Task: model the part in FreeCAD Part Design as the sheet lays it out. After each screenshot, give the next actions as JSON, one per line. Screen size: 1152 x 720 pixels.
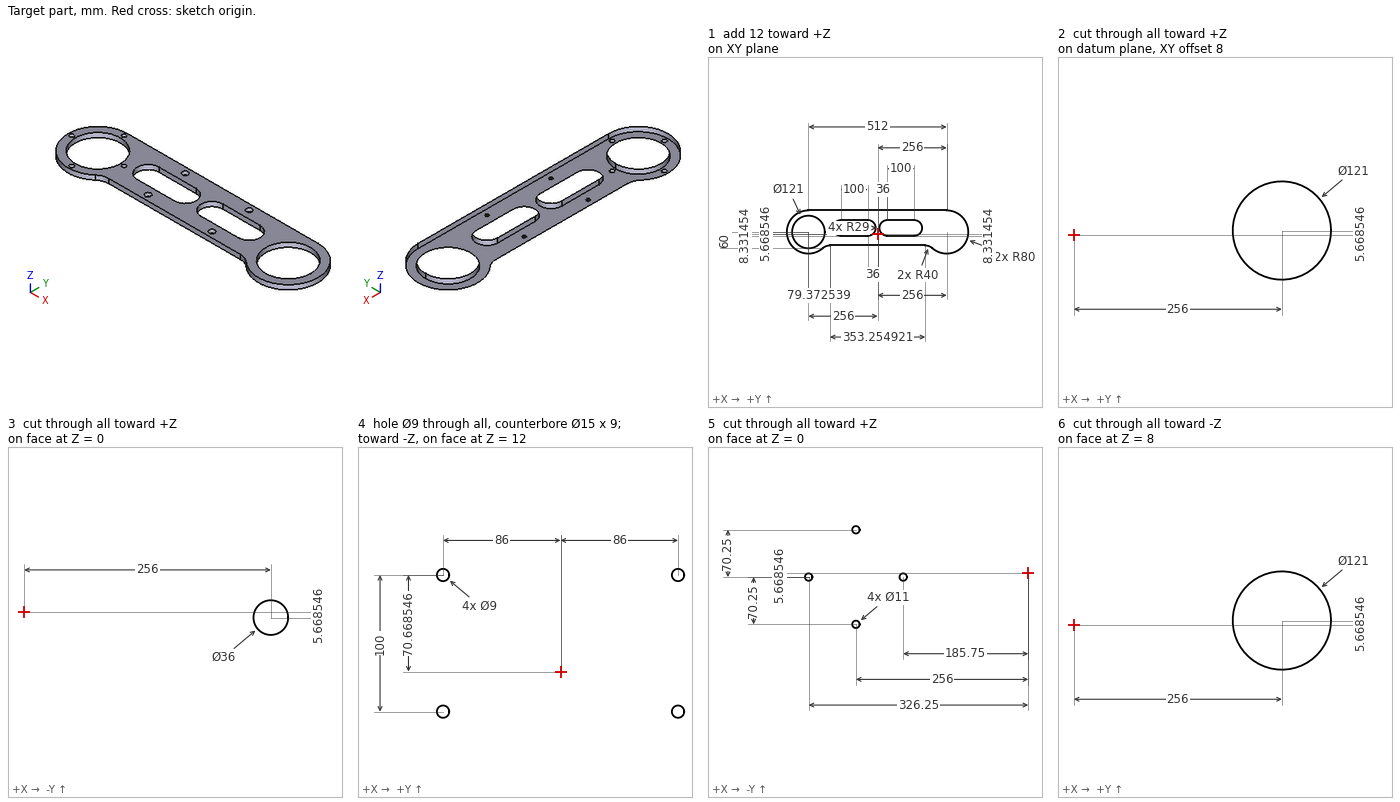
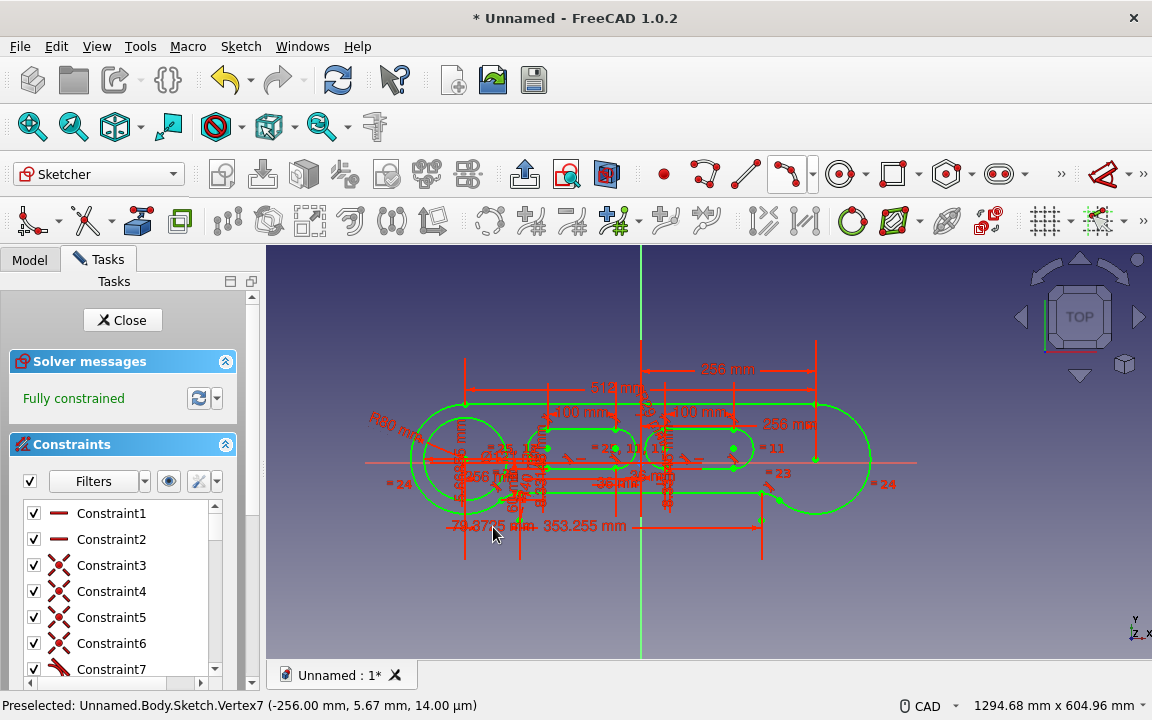
{"action": "left_click", "coordinate": [123, 320]}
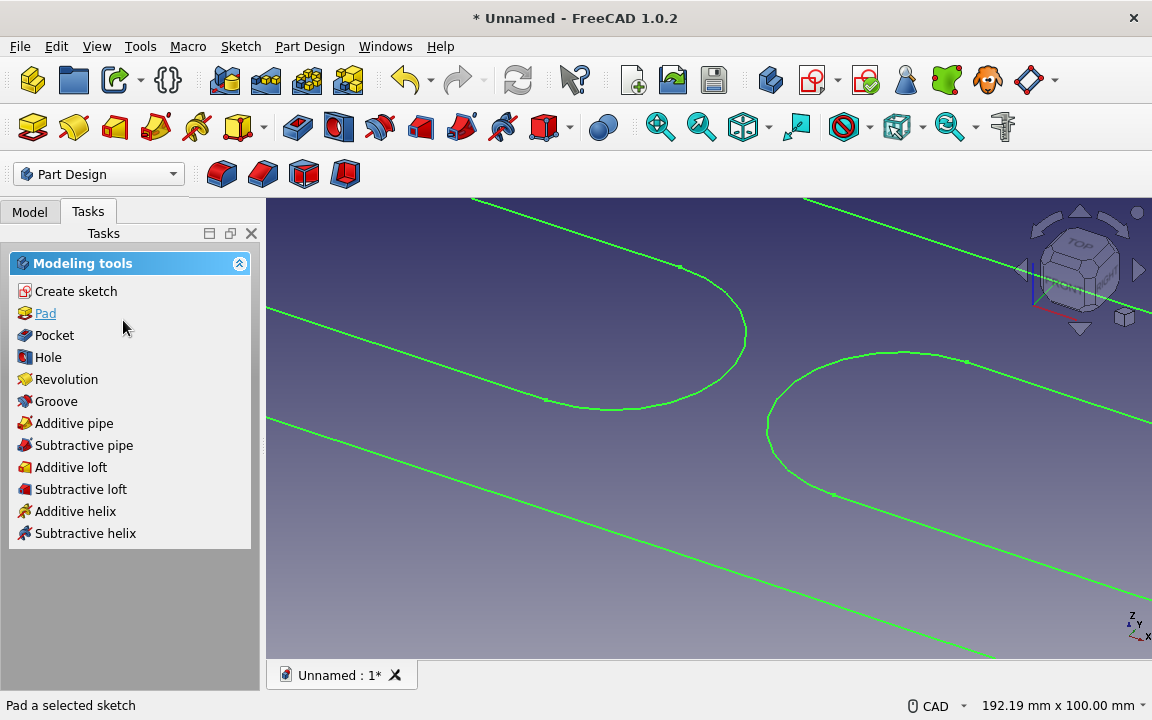
{"action": "left_click", "coordinate": [33, 128]}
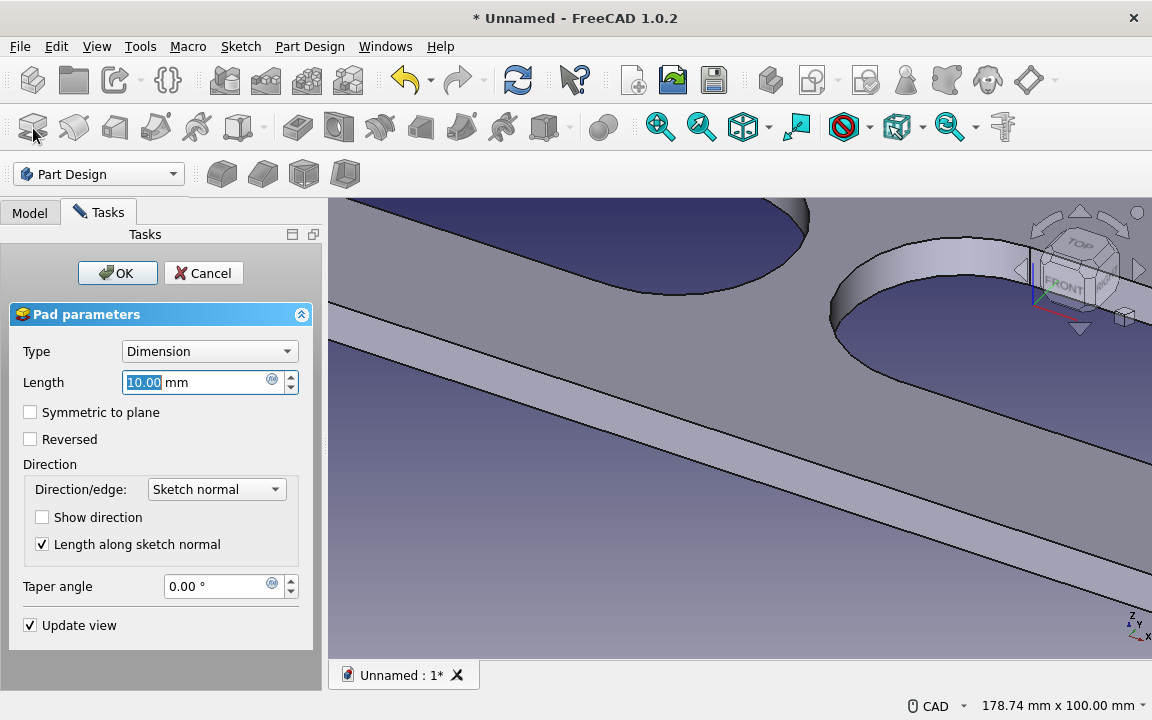
{"action": "type", "text": "12"}
{"action": "key", "text": "Tab"}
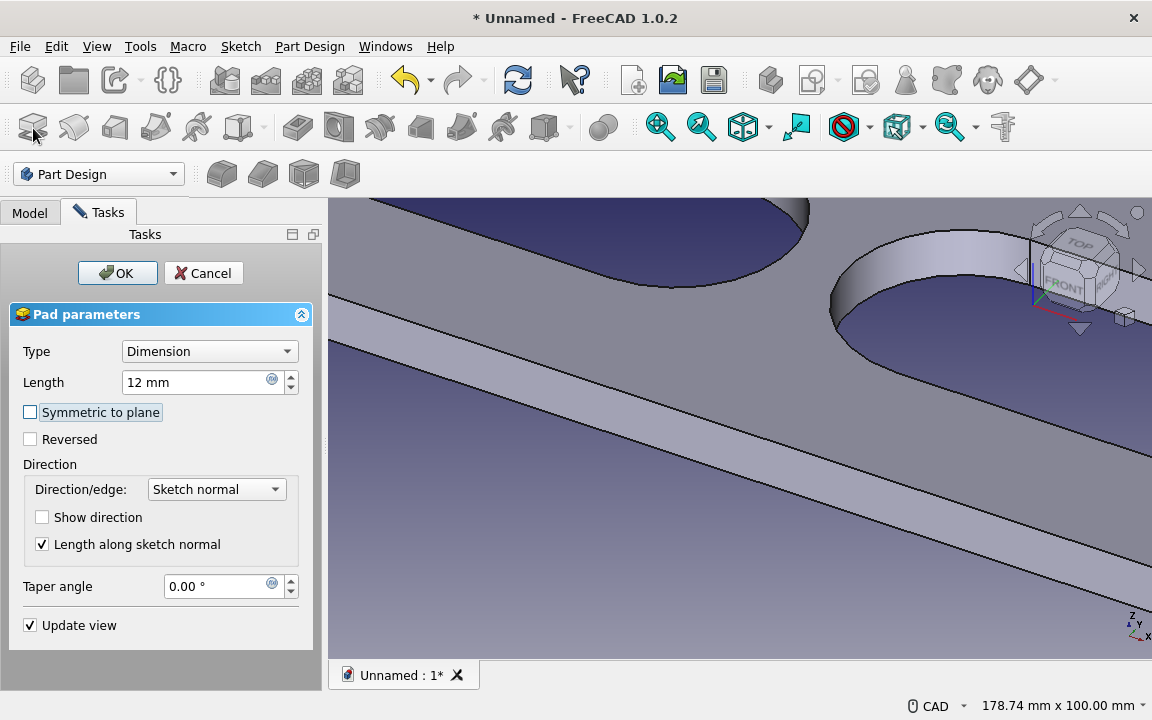
{"action": "left_click", "coordinate": [118, 273]}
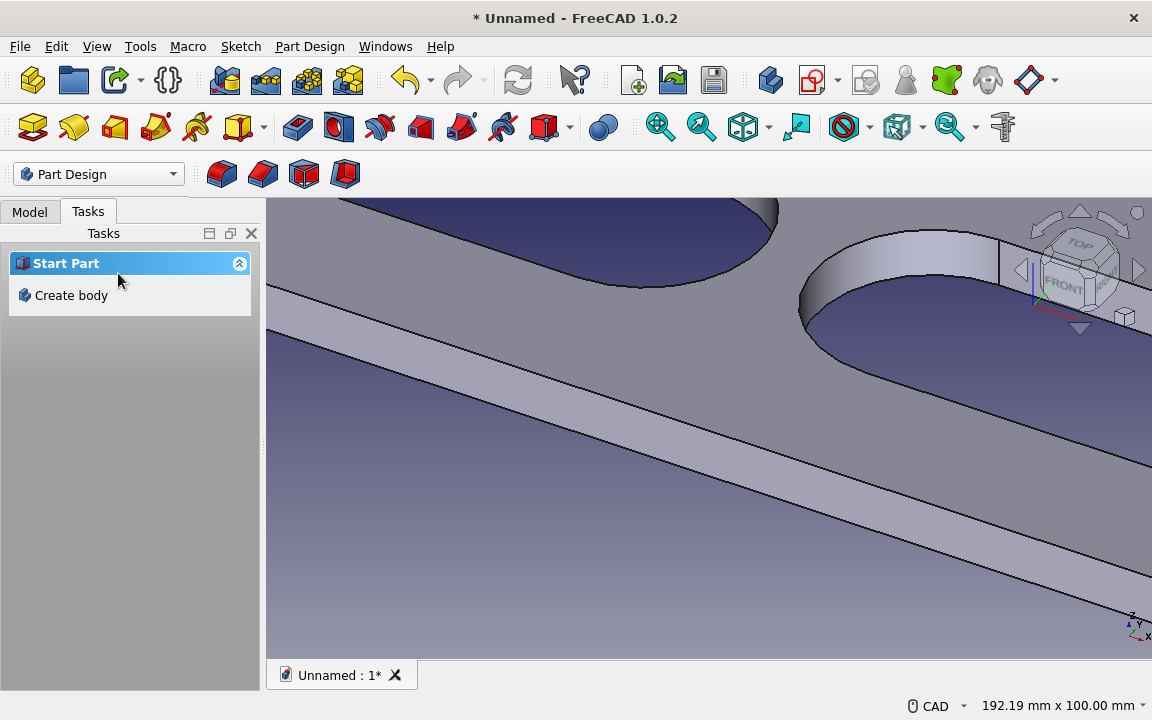
{"action": "left_click", "coordinate": [661, 128]}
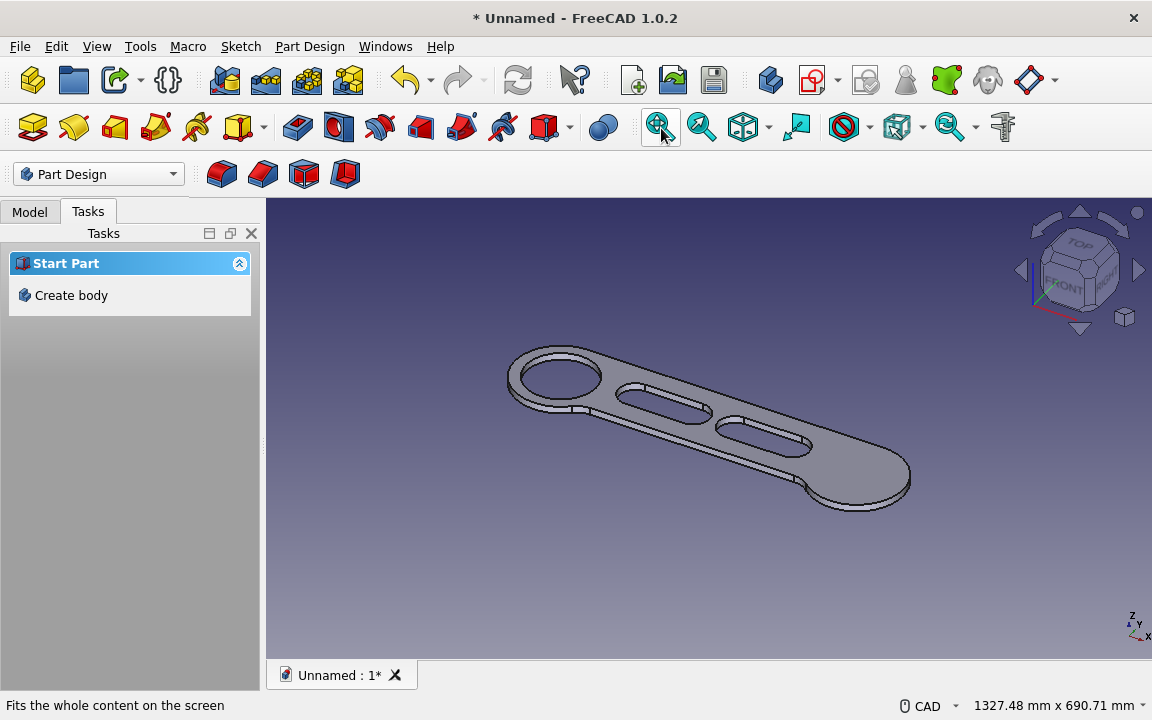
{"action": "left_click", "coordinate": [30, 212]}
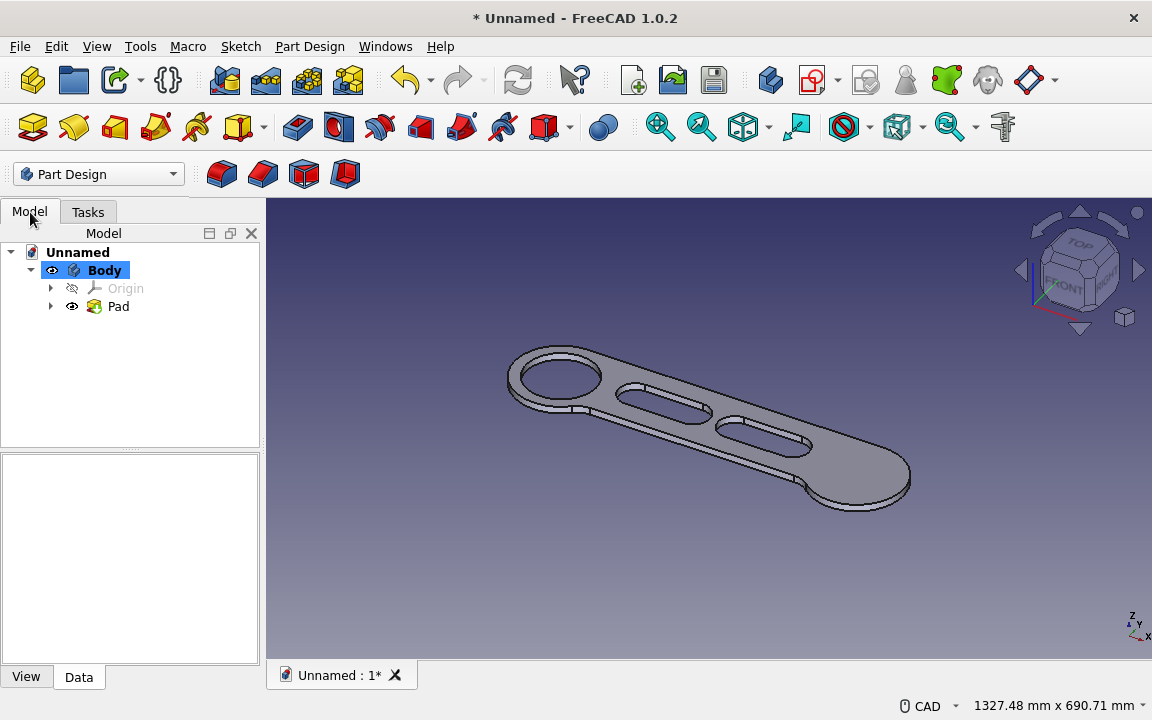
{"action": "left_click", "coordinate": [51, 288]}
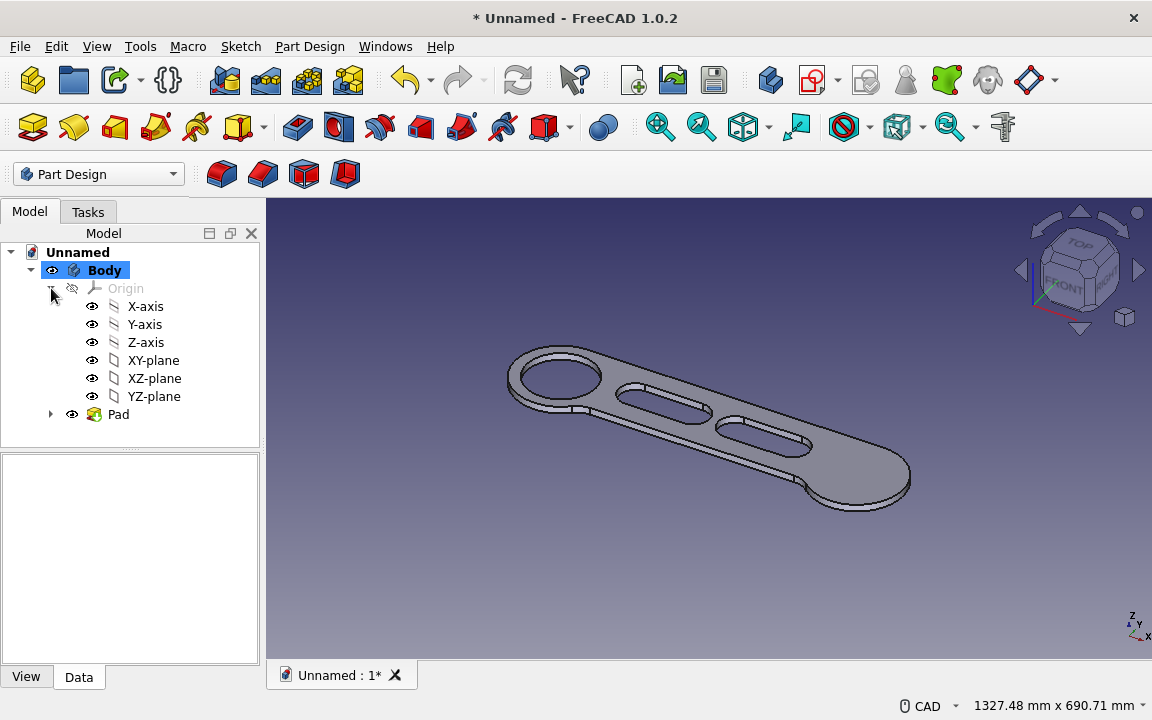
{"action": "left_click", "coordinate": [137, 360]}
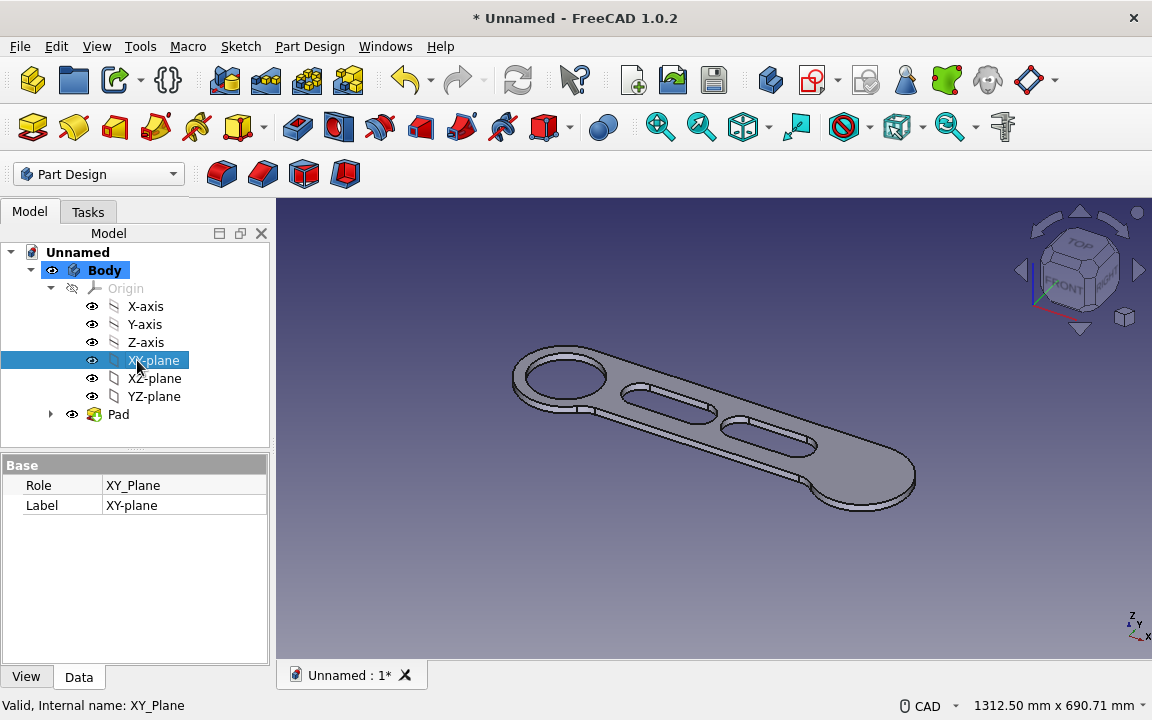
{"action": "left_click", "coordinate": [1028, 80]}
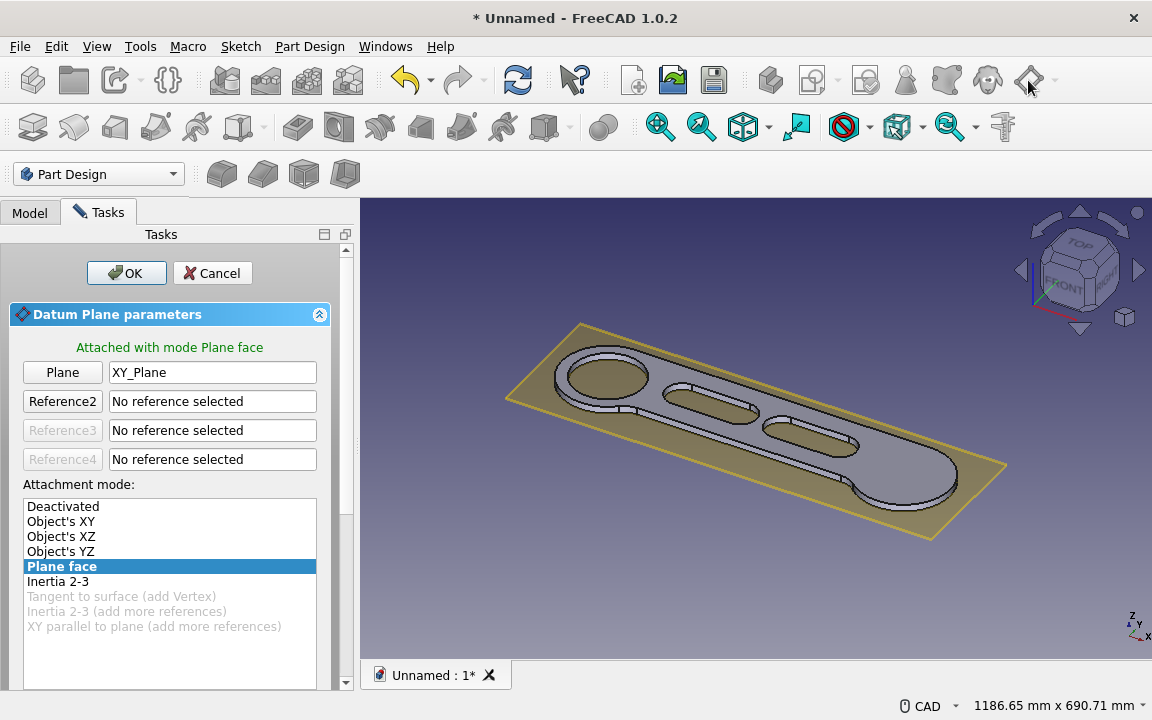
{"action": "scroll", "coordinate": [346, 467], "scroll_direction": "down", "scroll_amount": 4}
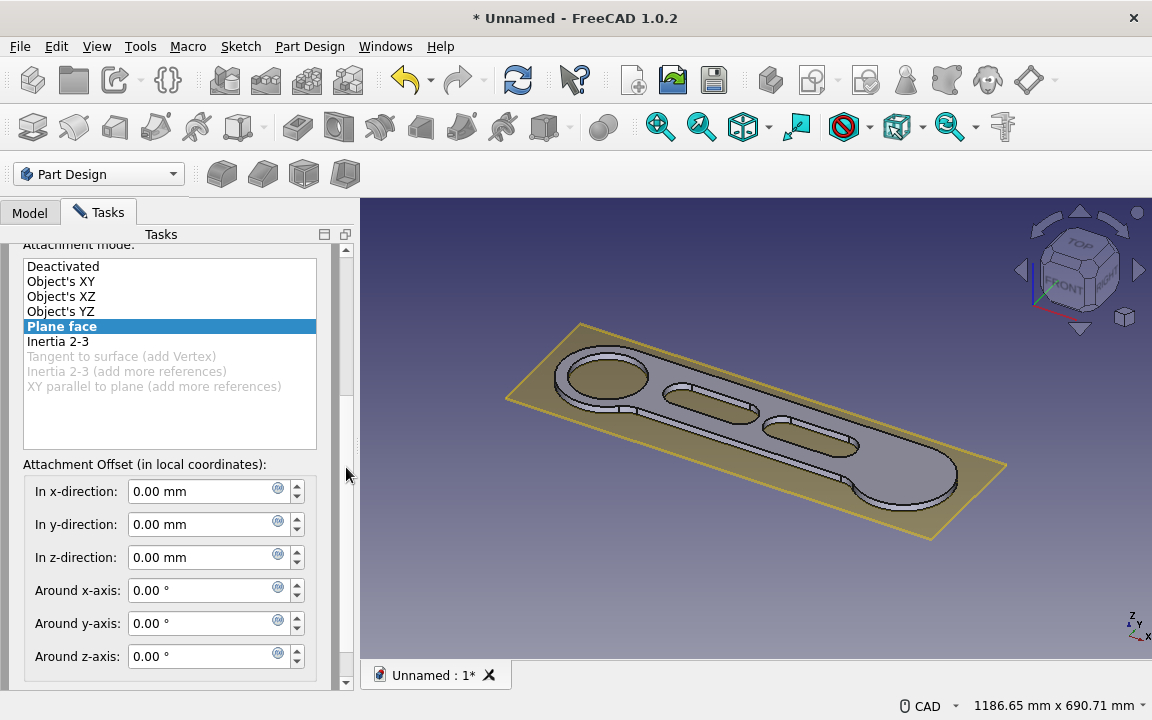
{"action": "triple_click", "coordinate": [210, 558]}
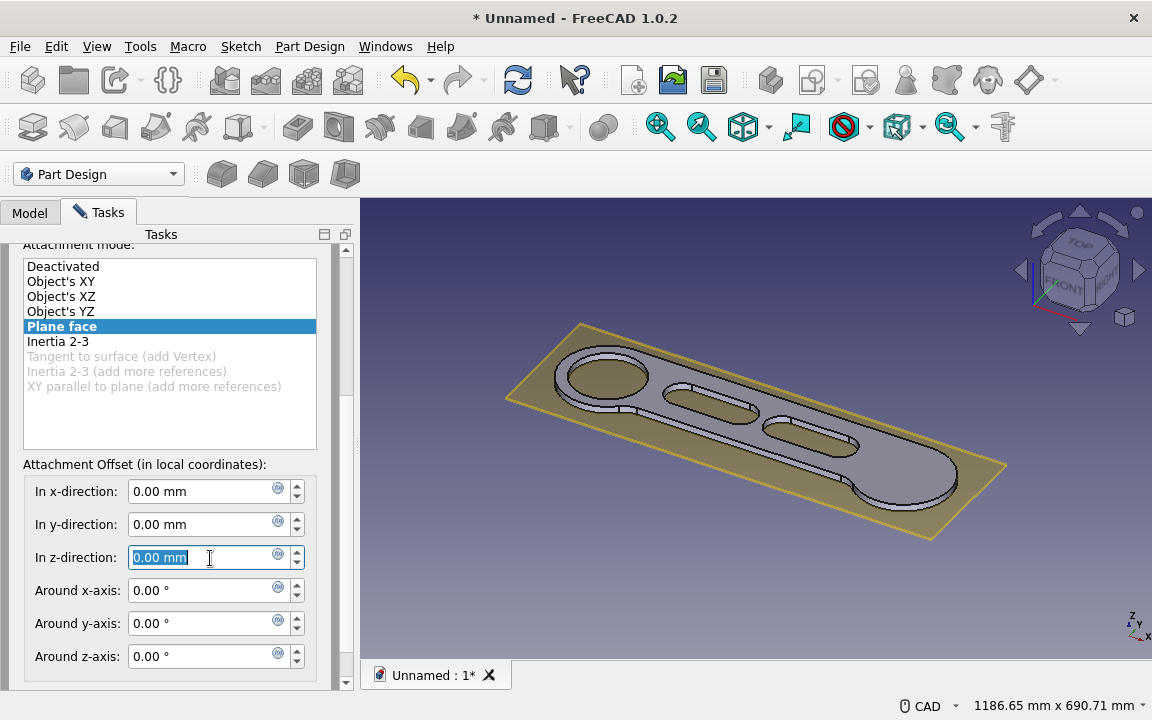
{"action": "type", "text": "8"}
{"action": "key", "text": "Tab"}